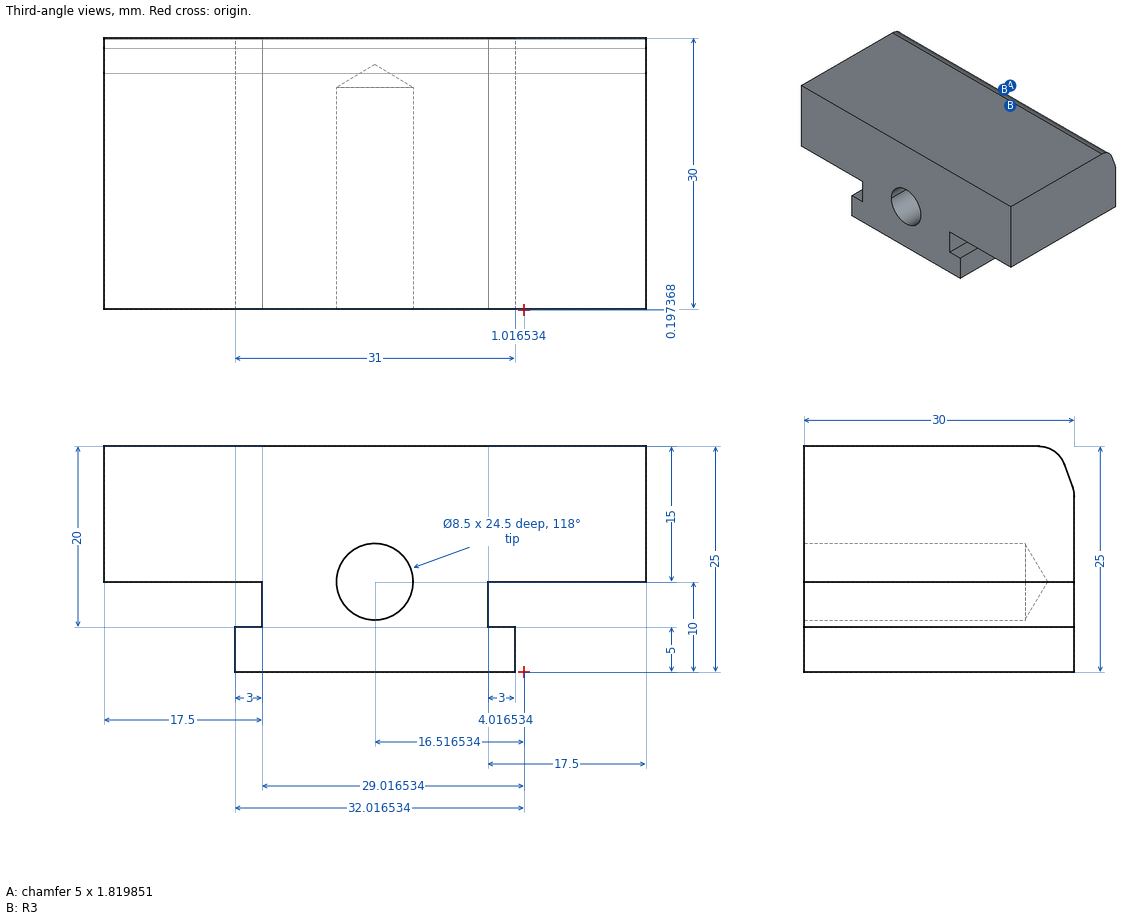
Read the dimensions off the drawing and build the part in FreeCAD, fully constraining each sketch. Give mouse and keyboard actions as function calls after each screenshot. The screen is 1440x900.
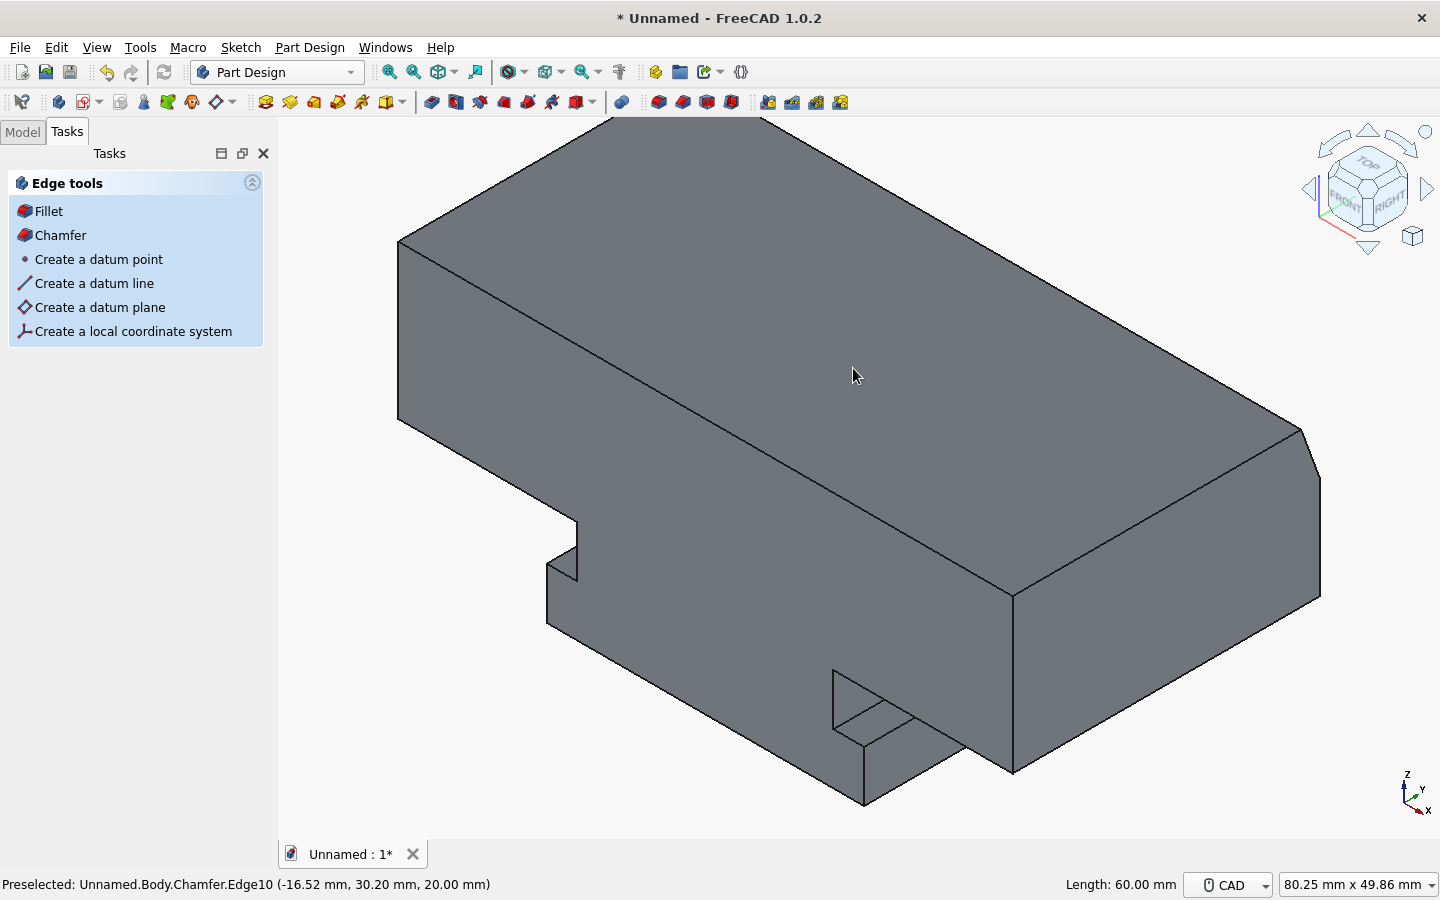
click(390, 72)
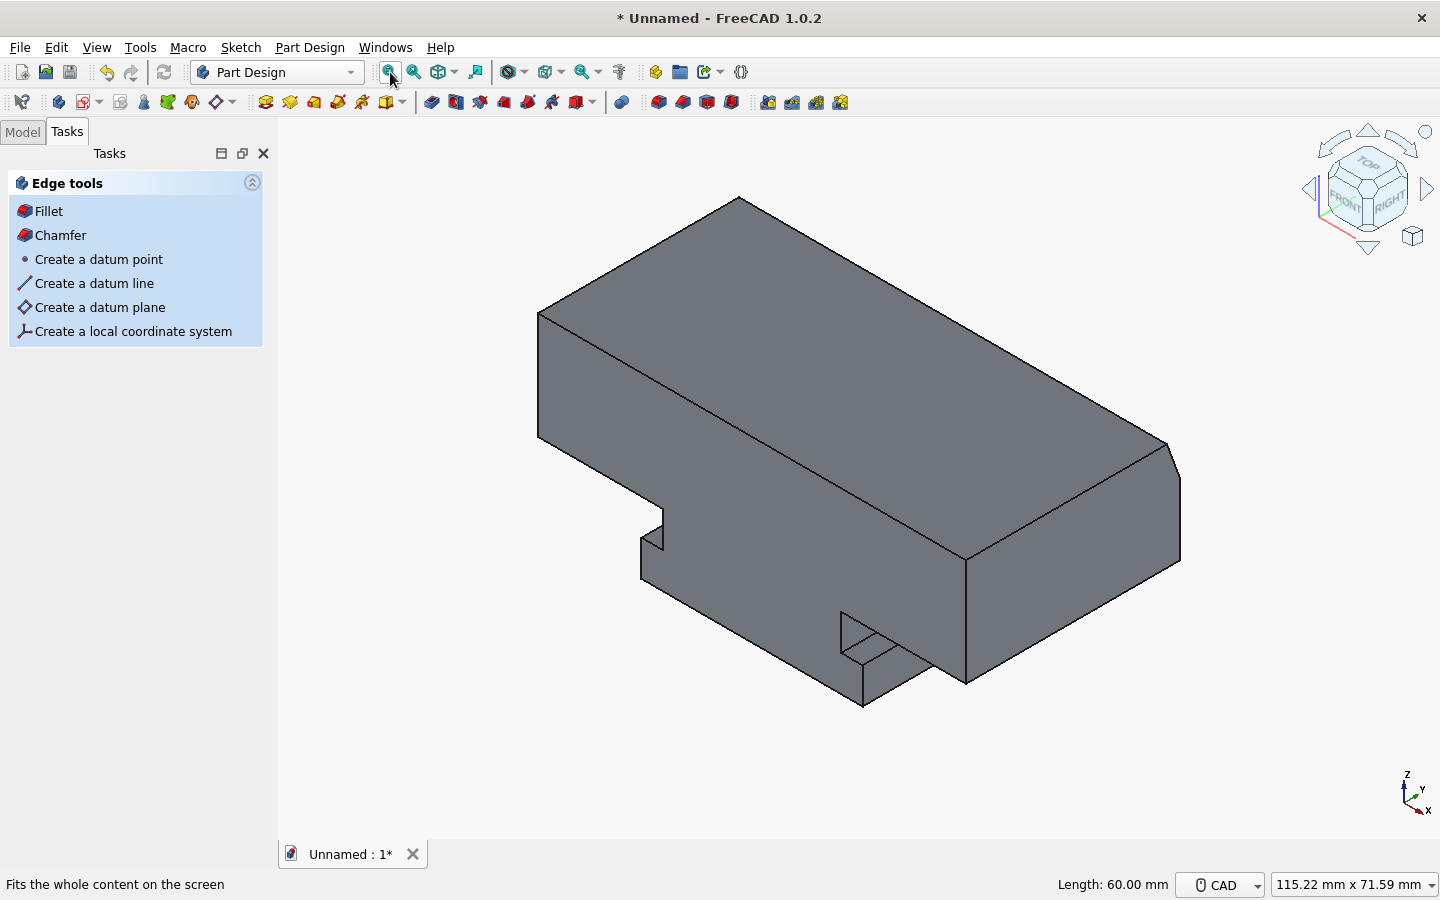
key(2)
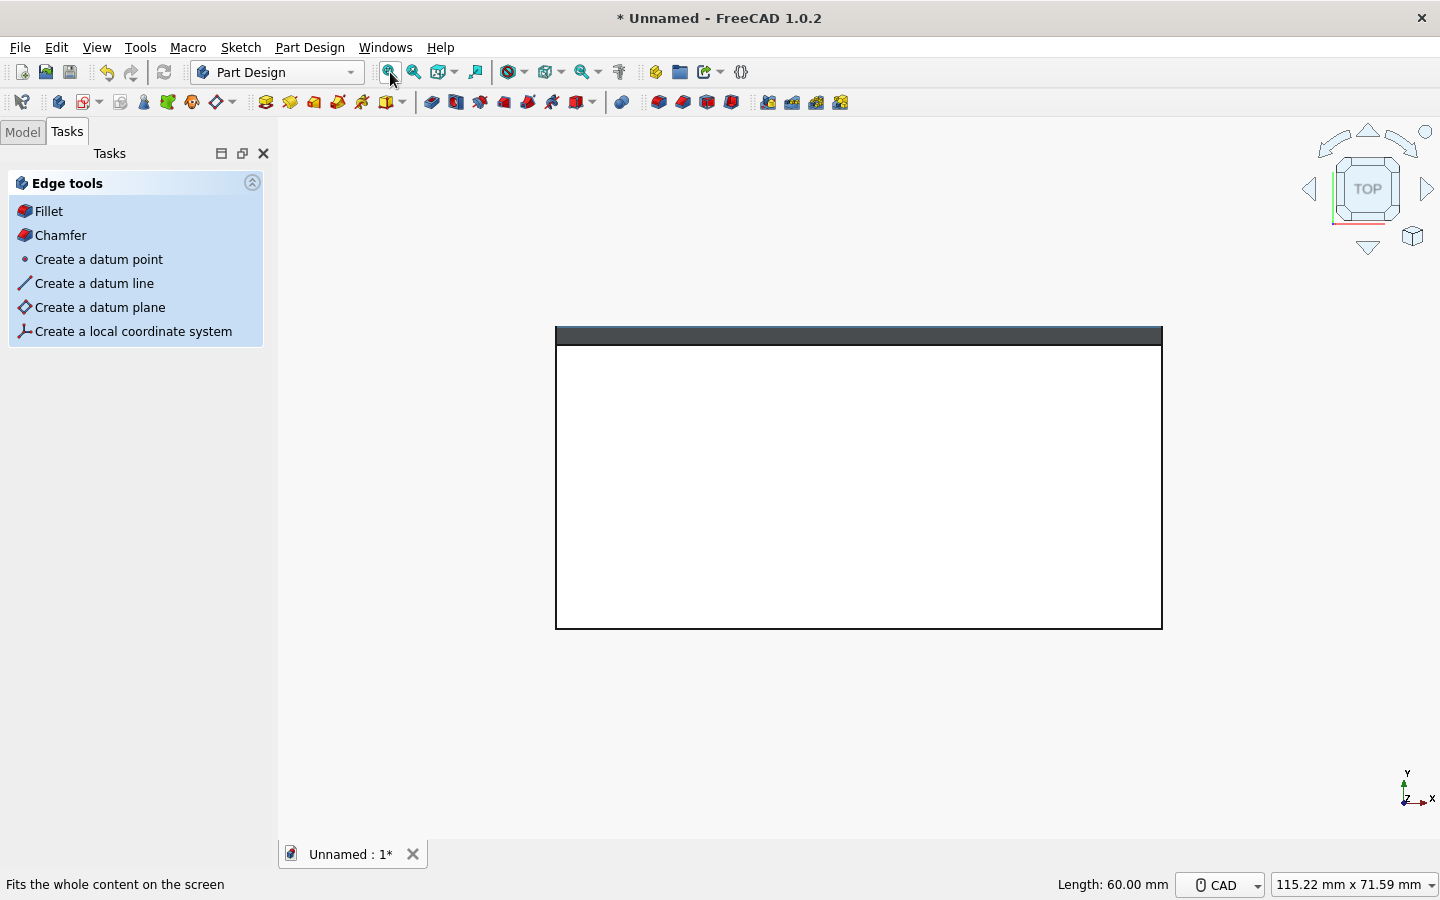
click(859, 344, ctrl)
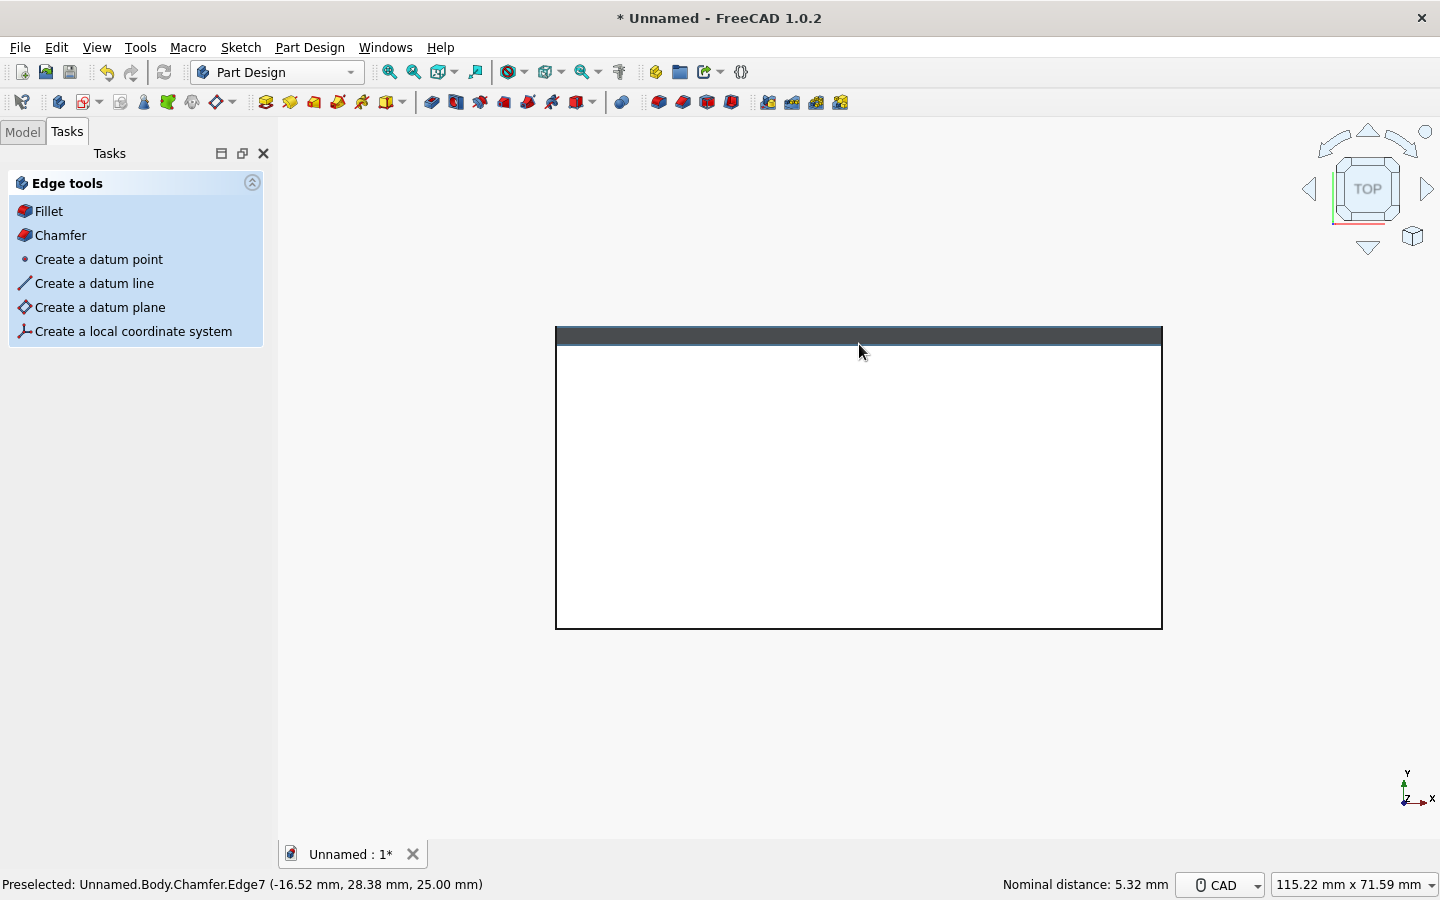
click(660, 102)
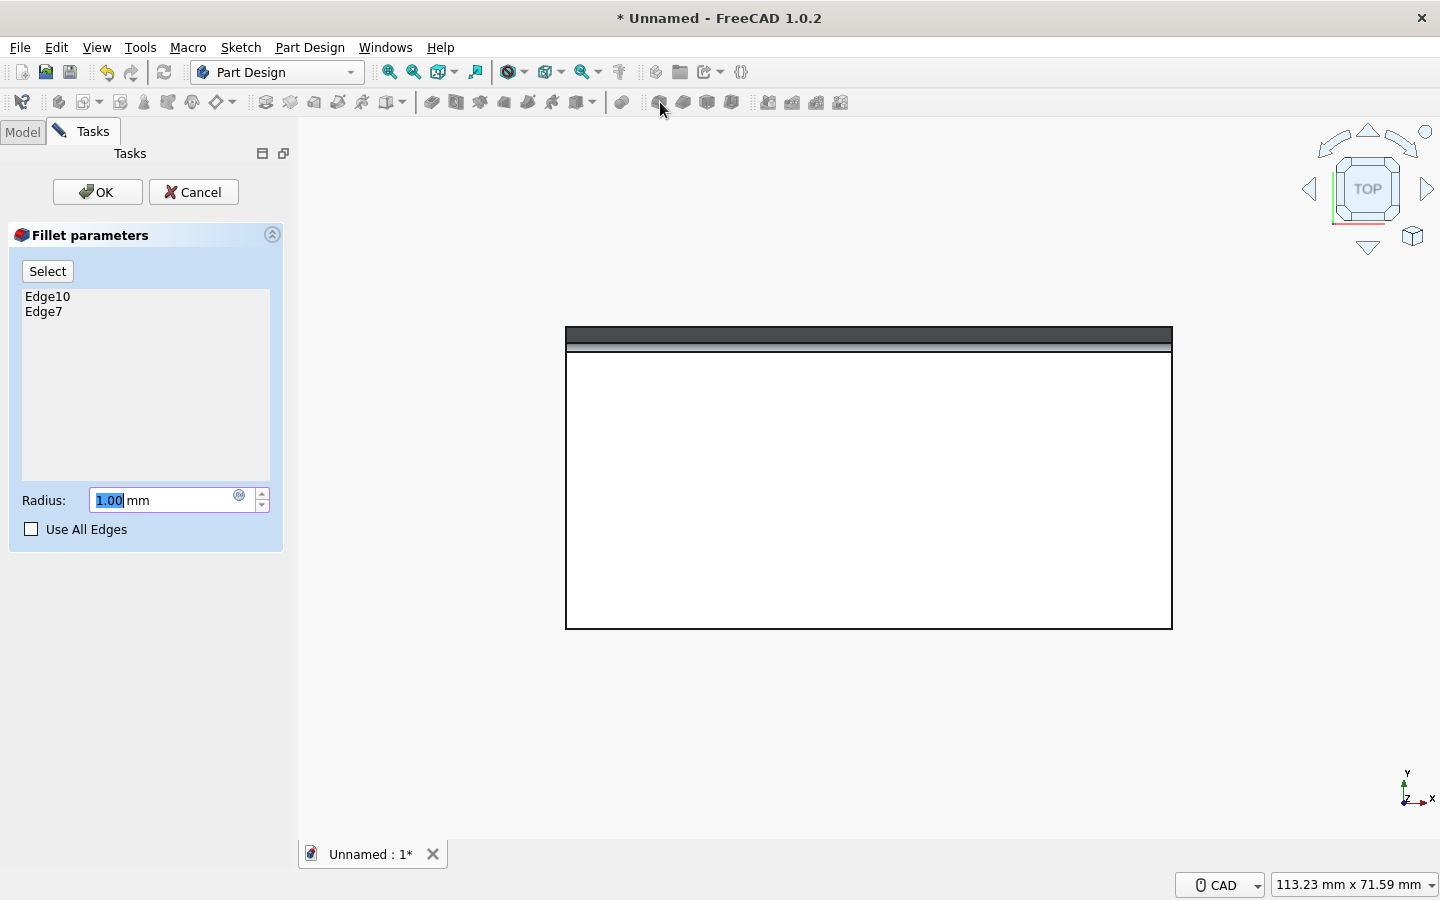
text(3)
key(Tab)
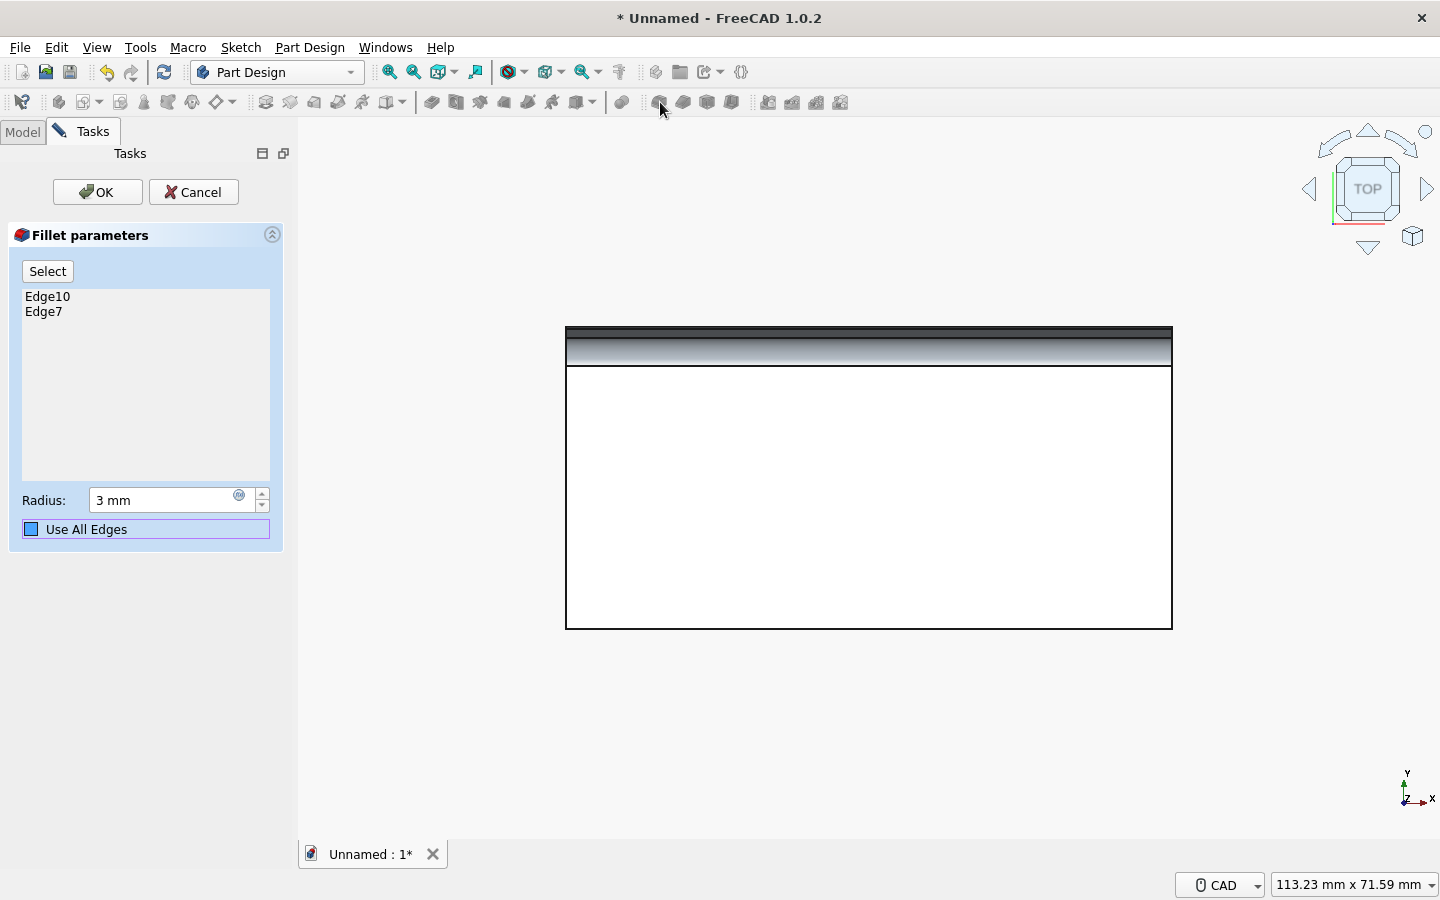
click(98, 192)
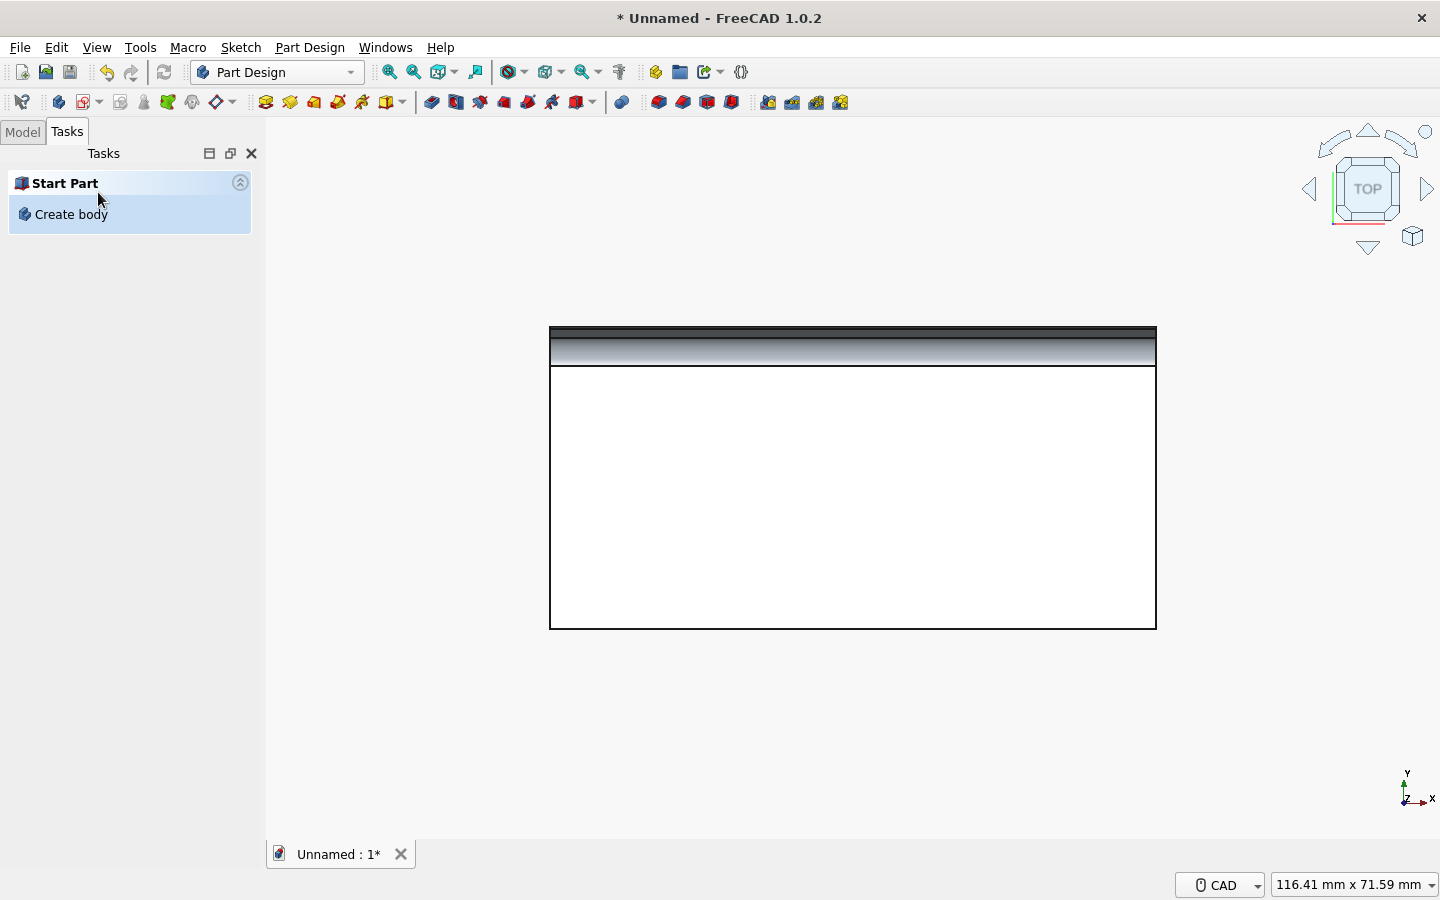
key(0)